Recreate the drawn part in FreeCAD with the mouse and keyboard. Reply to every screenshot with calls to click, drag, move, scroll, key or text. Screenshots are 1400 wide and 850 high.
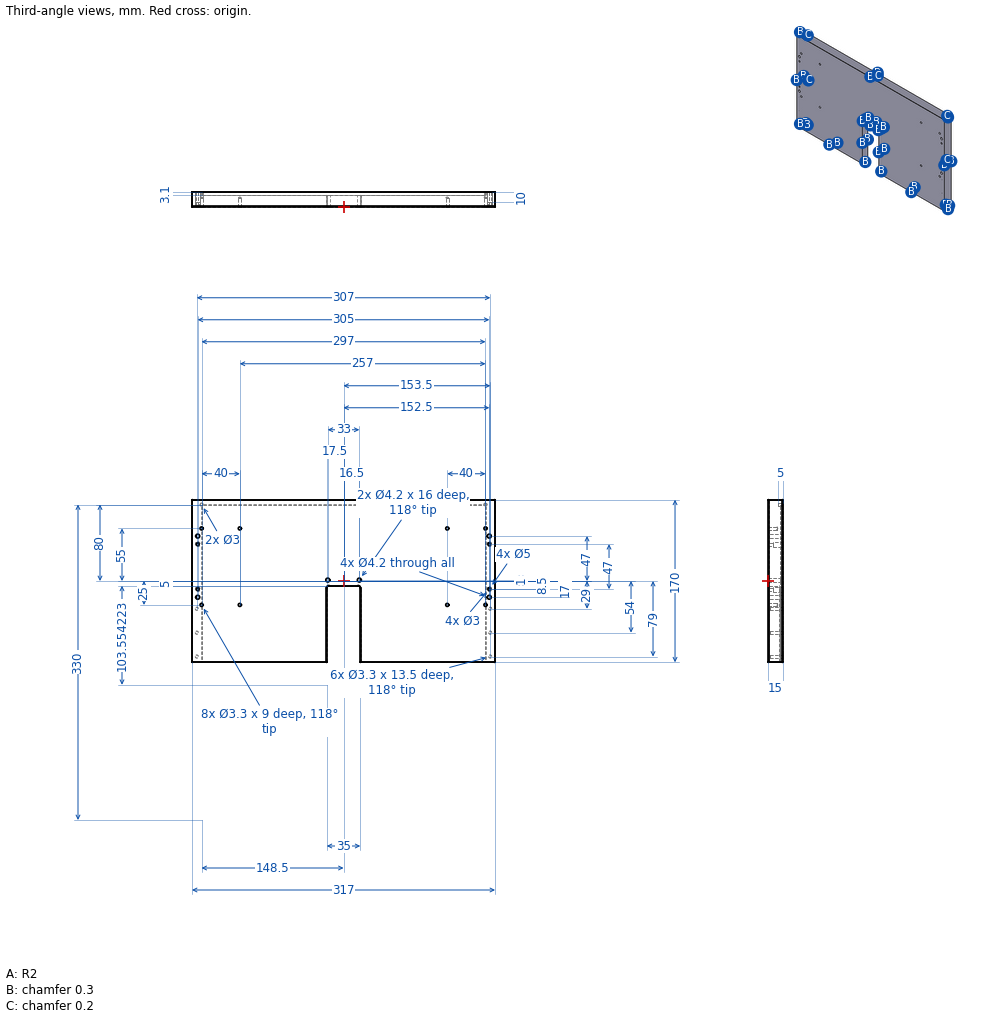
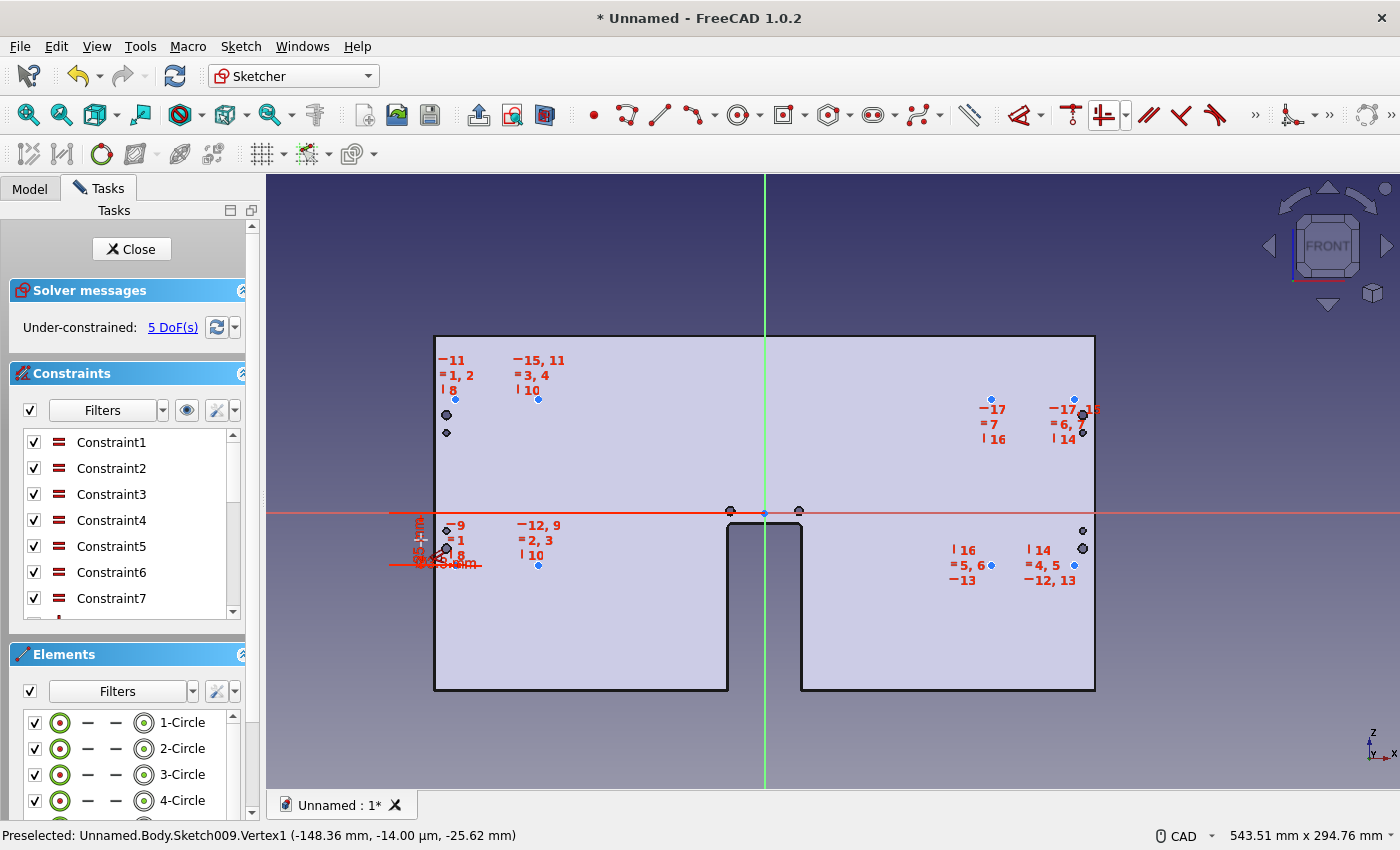
click(455, 400)
click(421, 456)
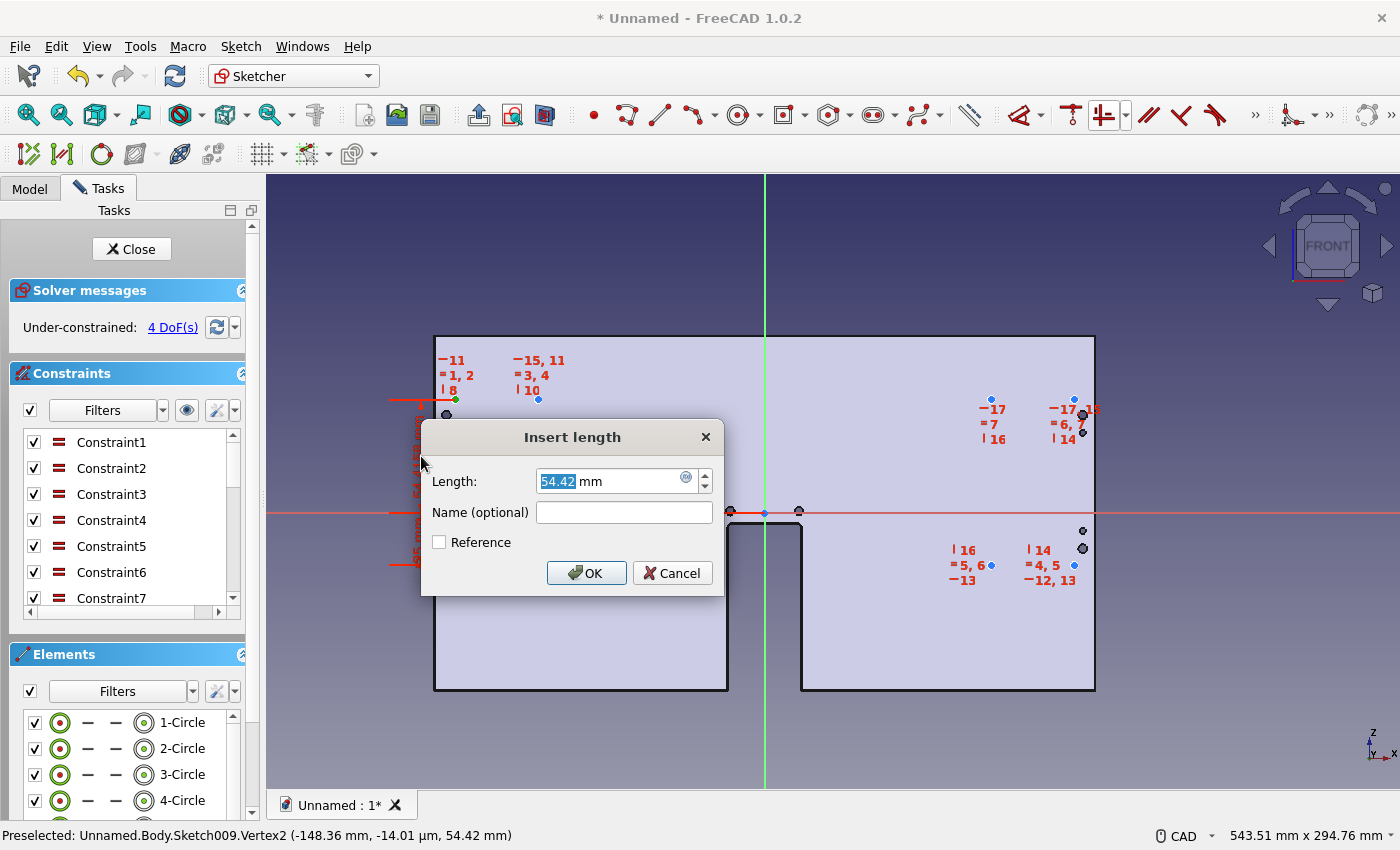
text(55)
key(Return)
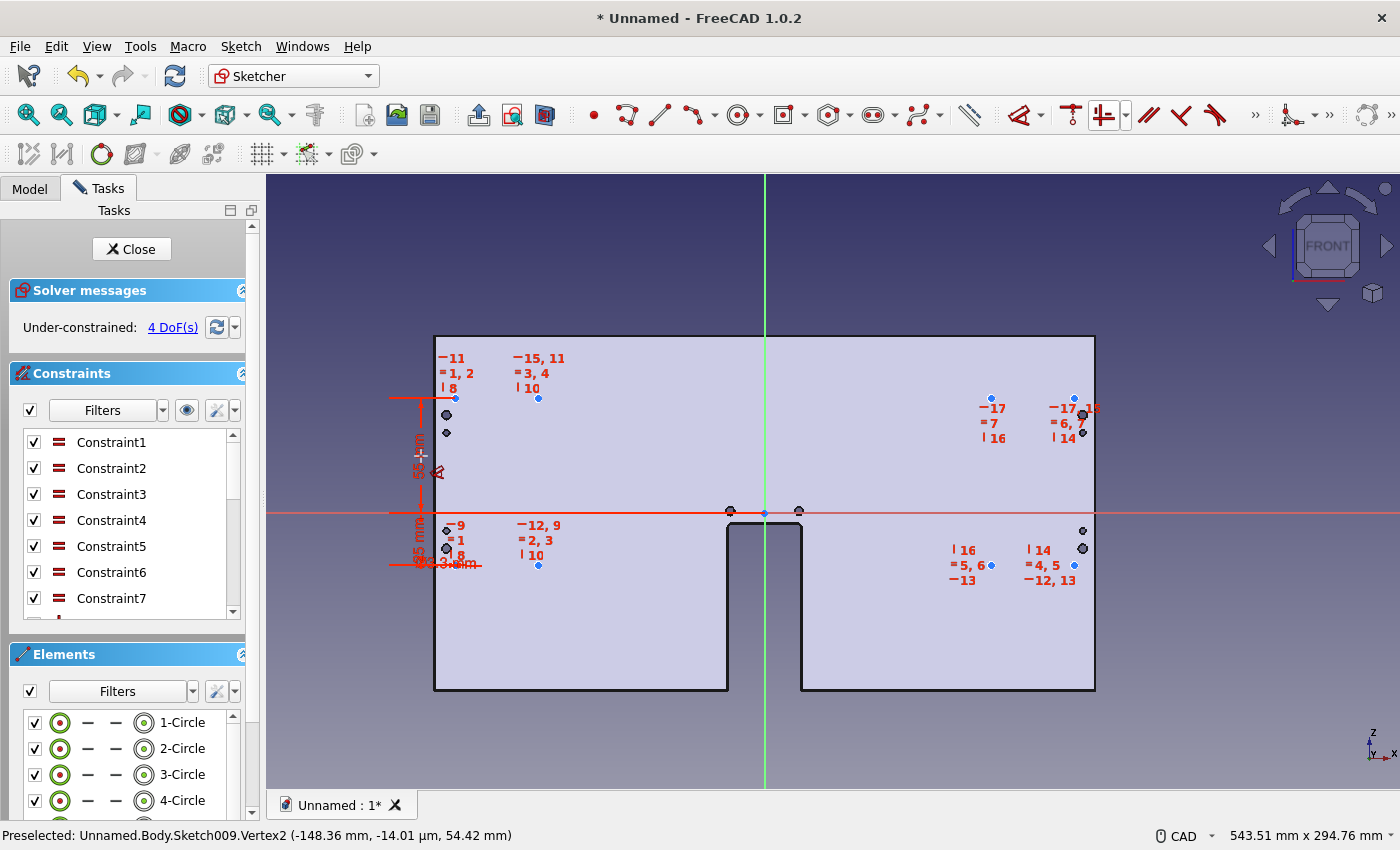
click(455, 565)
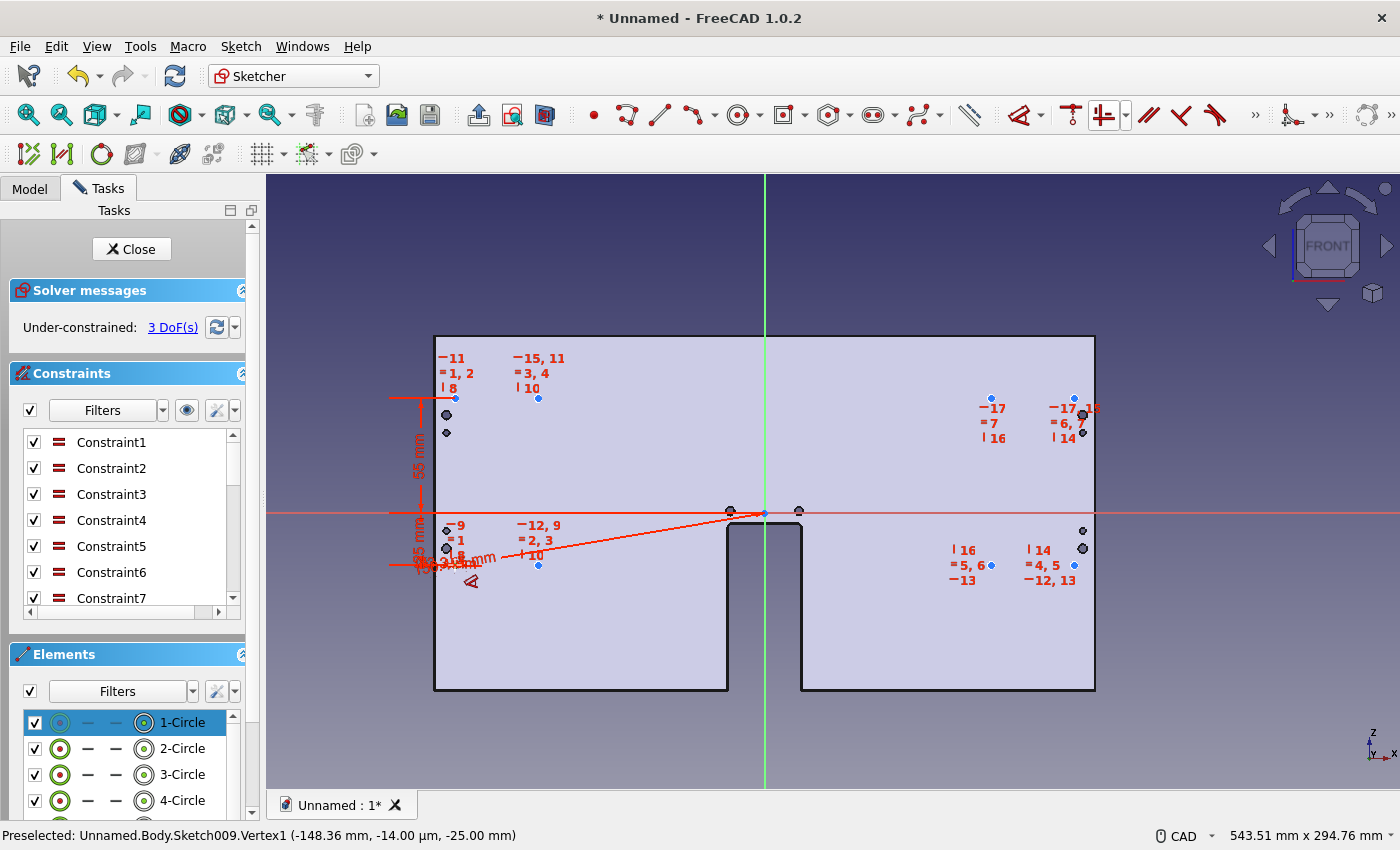
click(538, 565)
click(497, 599)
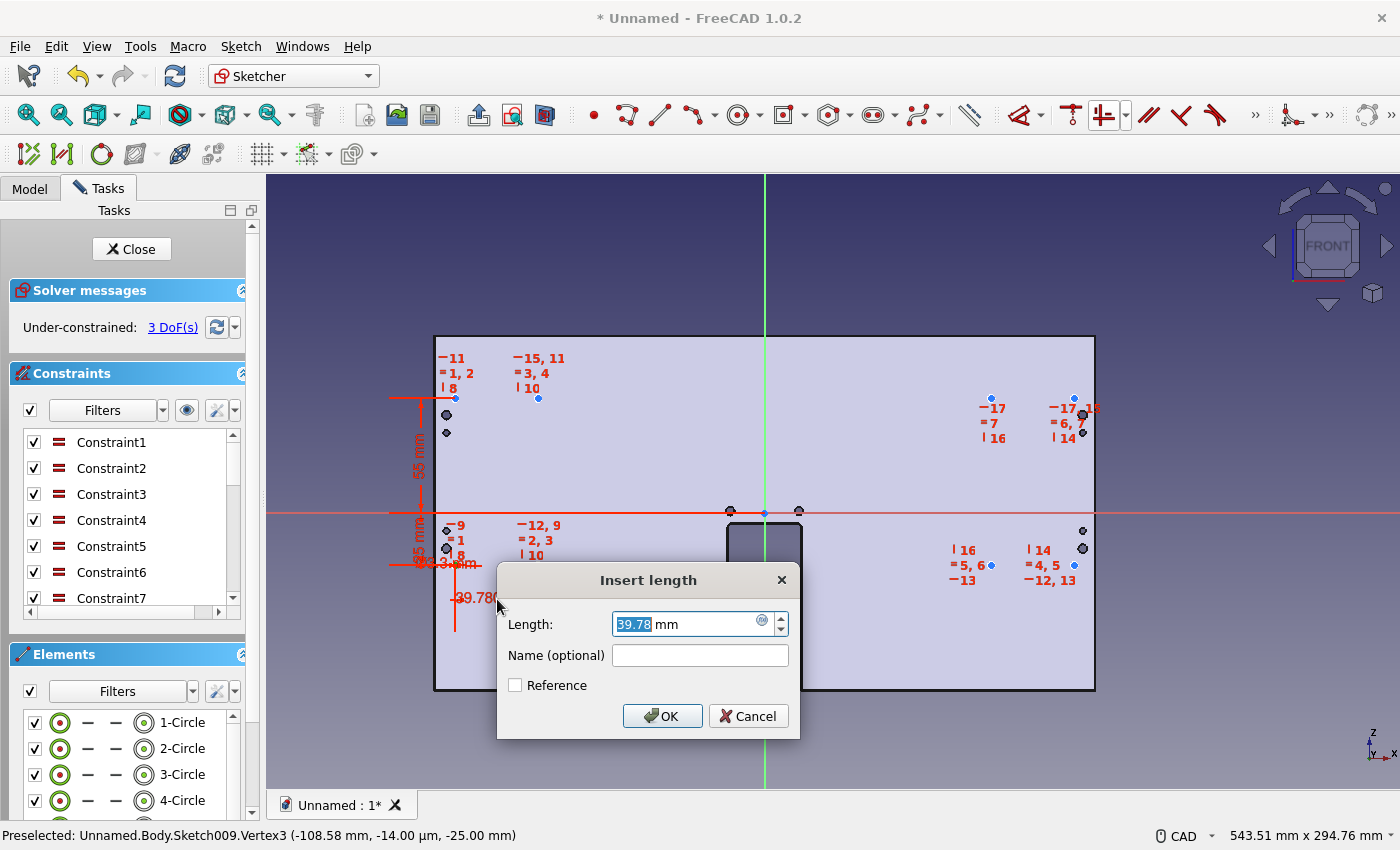
text(40)
key(Return)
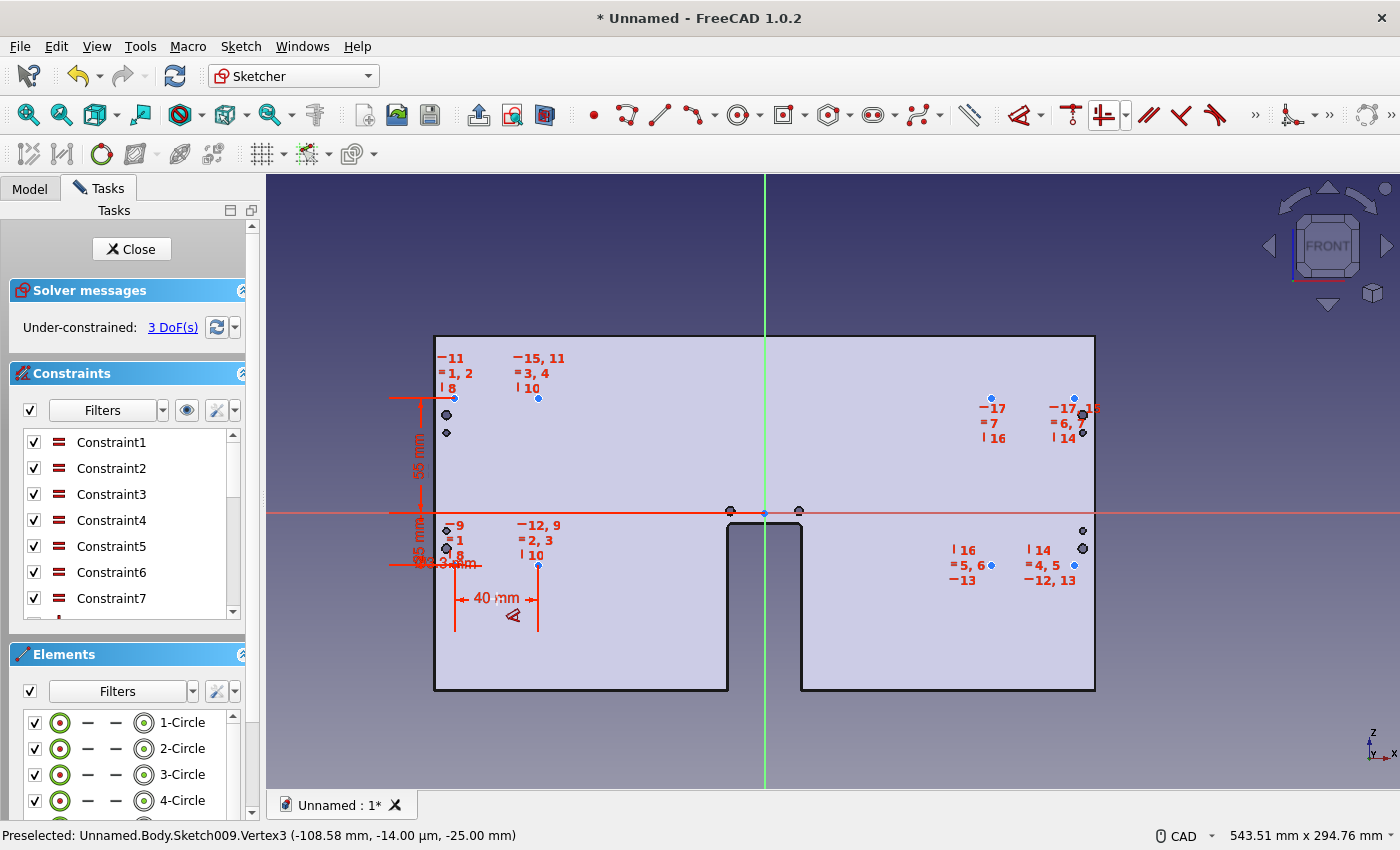
click(1074, 565)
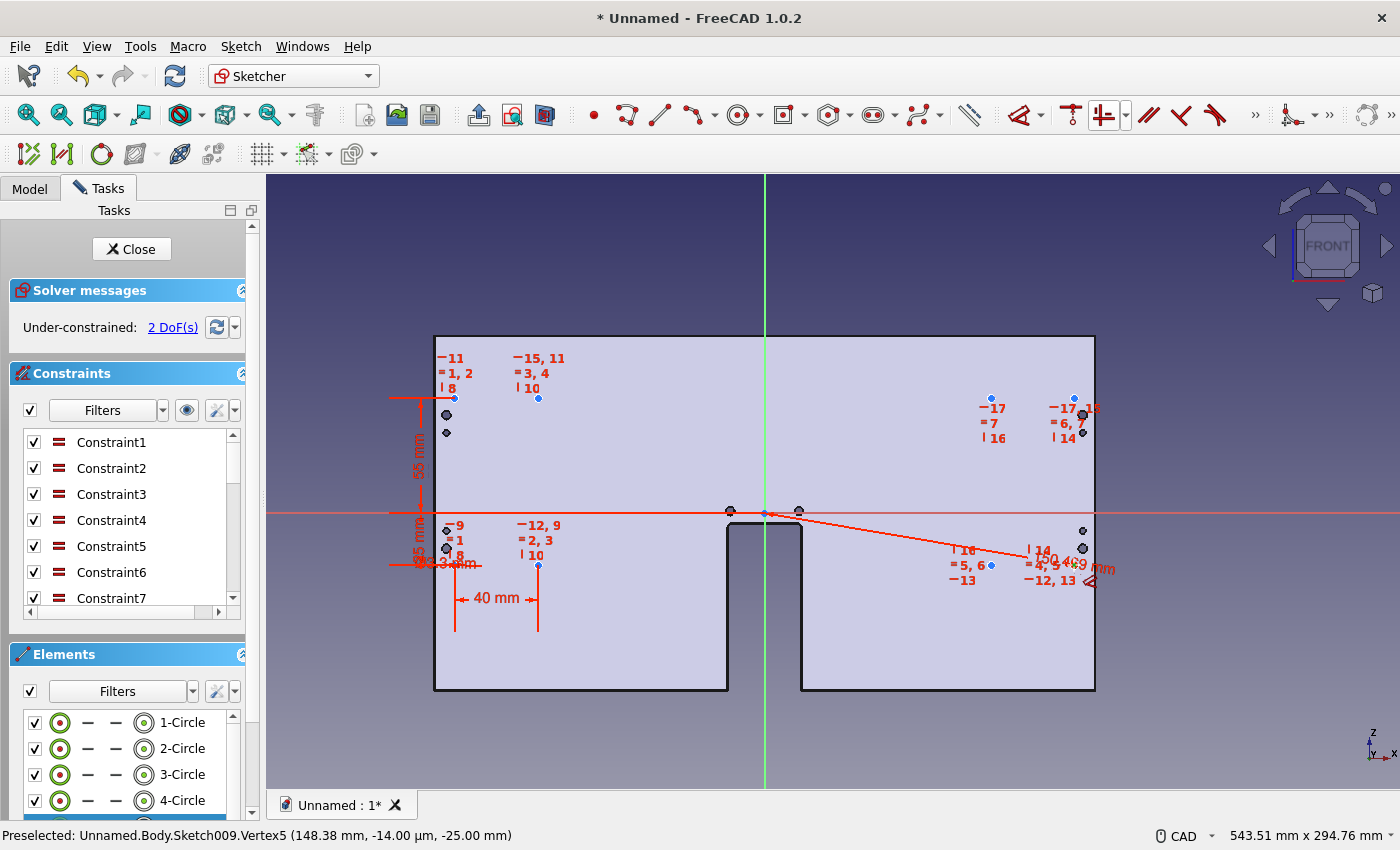
click(991, 565)
click(1033, 599)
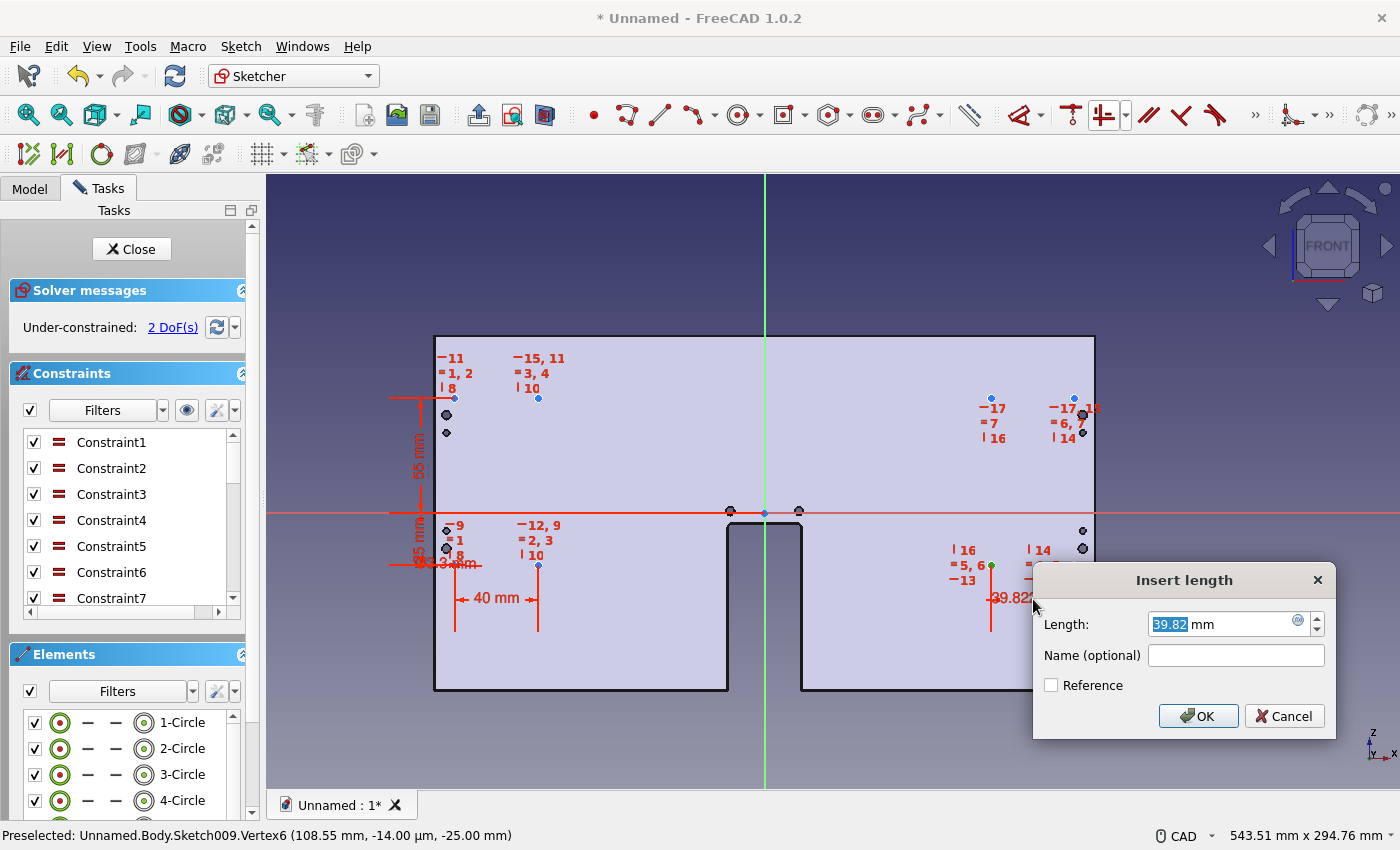
text(40)
key(Return)